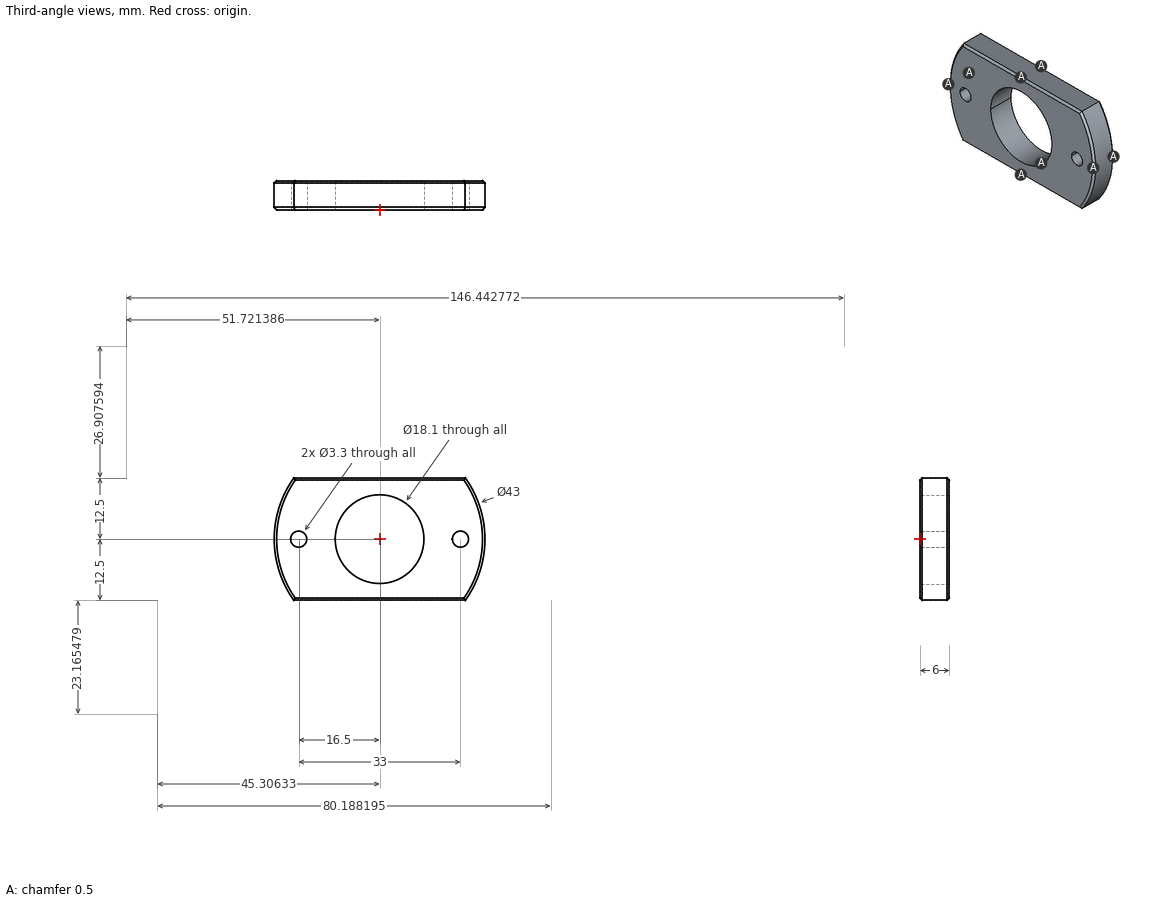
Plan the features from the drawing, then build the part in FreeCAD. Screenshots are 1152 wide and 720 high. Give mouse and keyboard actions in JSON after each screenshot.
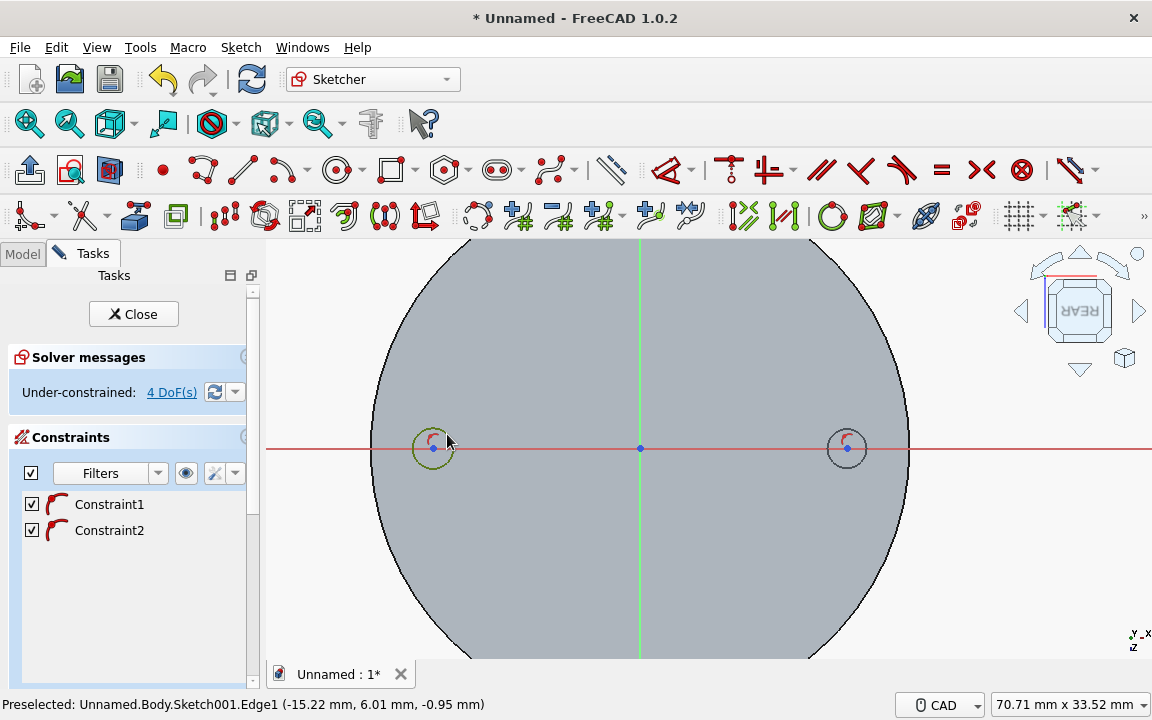
{"action": "left_click", "coordinate": [861, 435]}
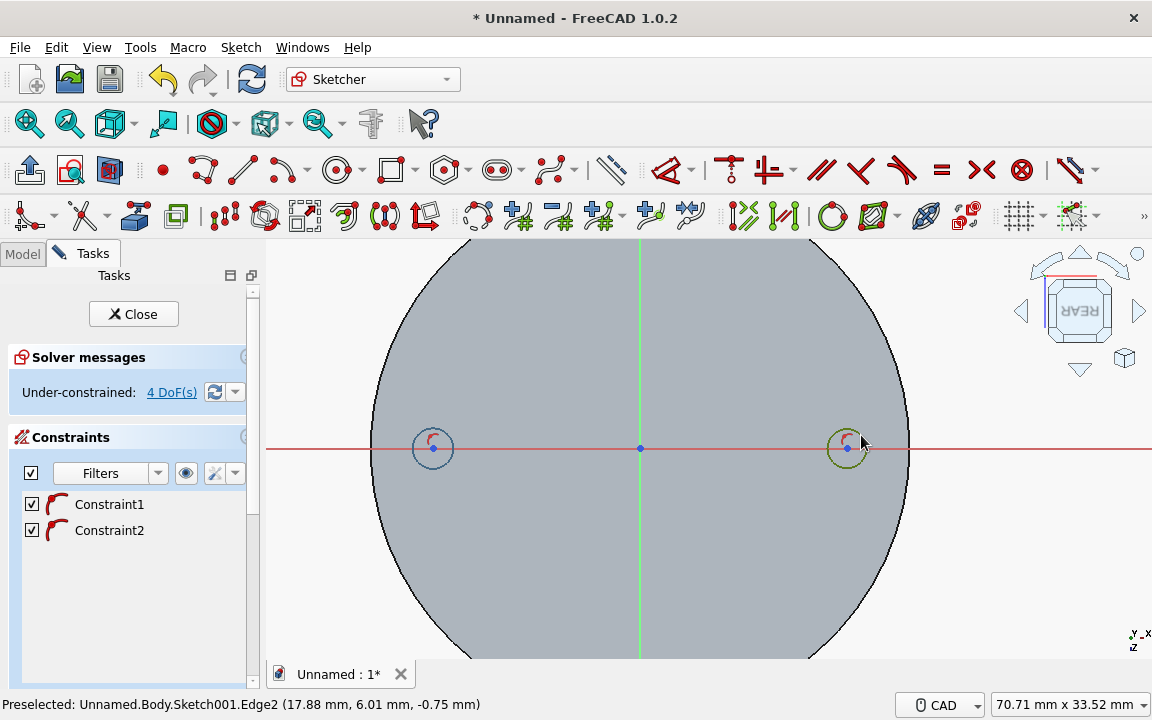
{"action": "left_click", "coordinate": [942, 170]}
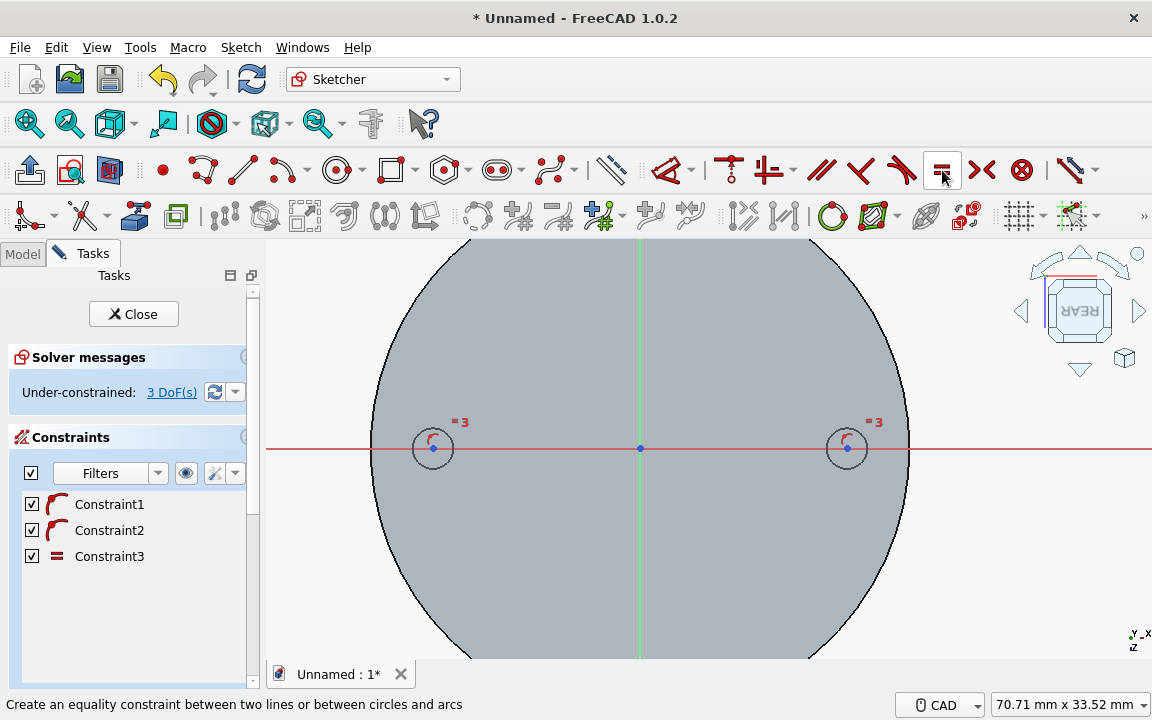
{"action": "left_click", "coordinate": [666, 170]}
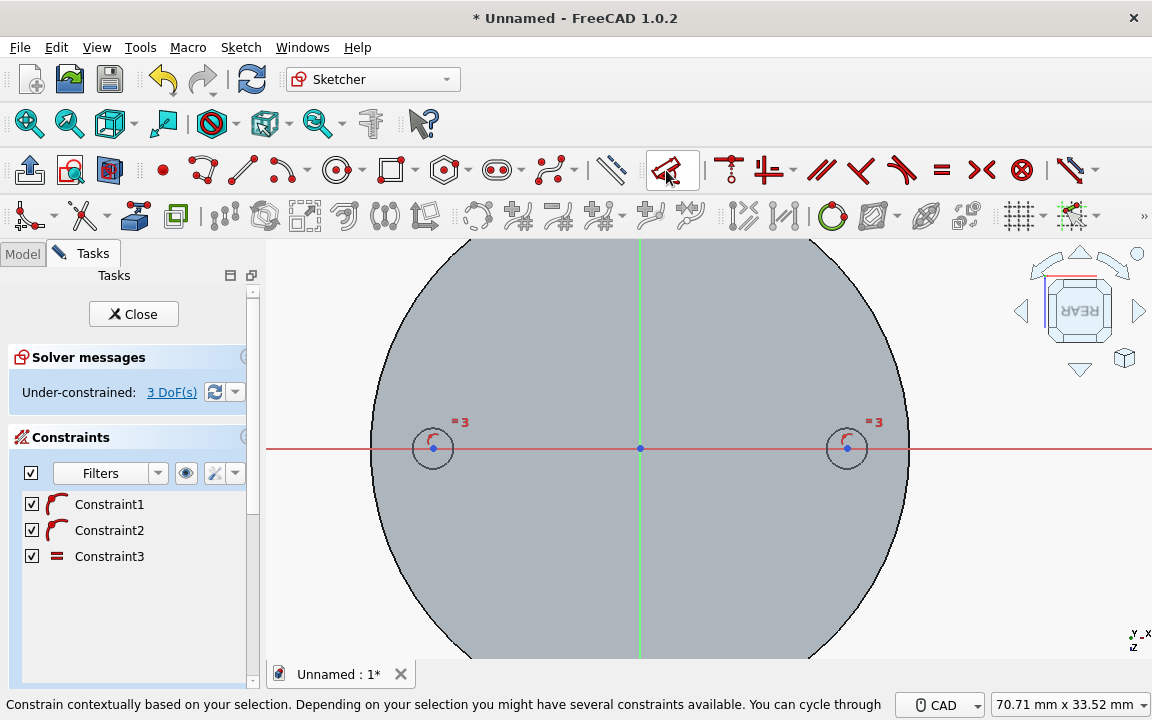
{"action": "left_click", "coordinate": [447, 434]}
{"action": "left_click", "coordinate": [469, 411]}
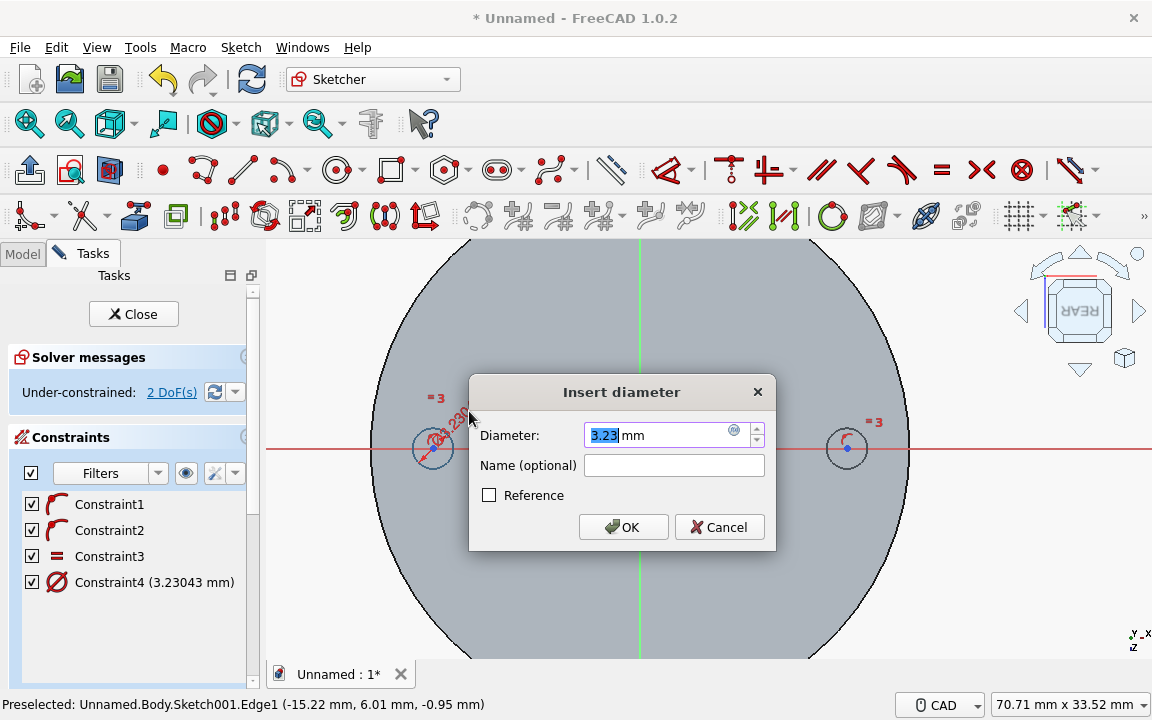
{"action": "type", "text": "3.3"}
{"action": "key", "text": "Return"}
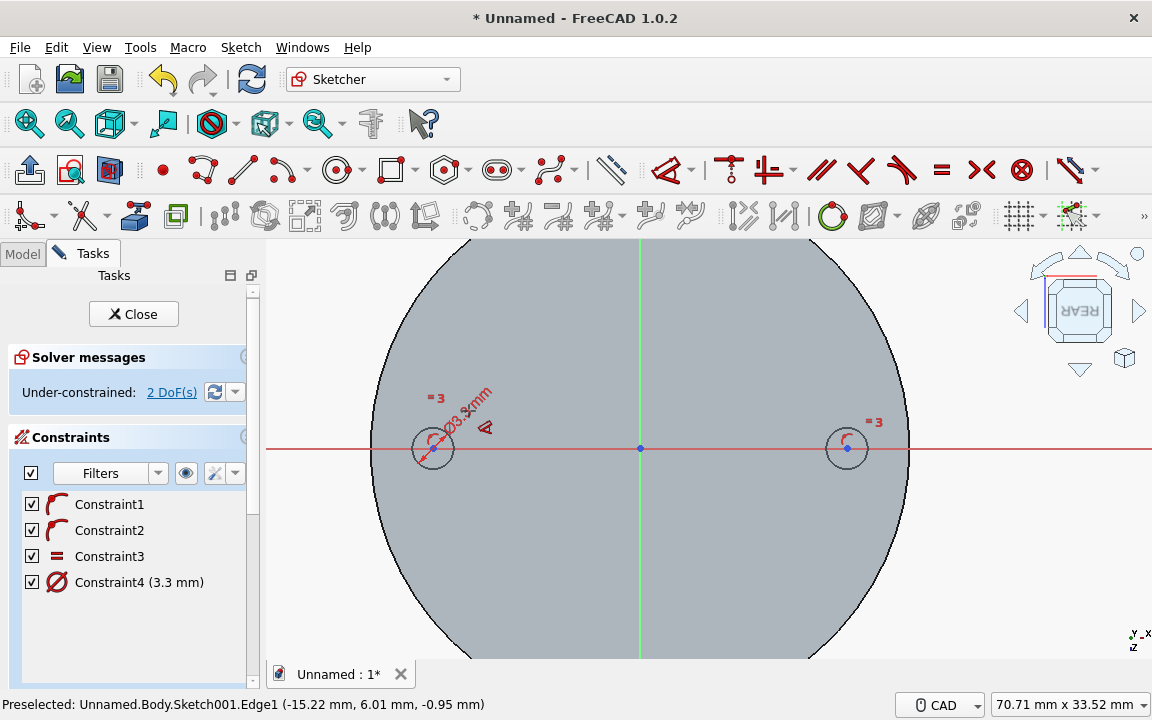
{"action": "left_click", "coordinate": [433, 449]}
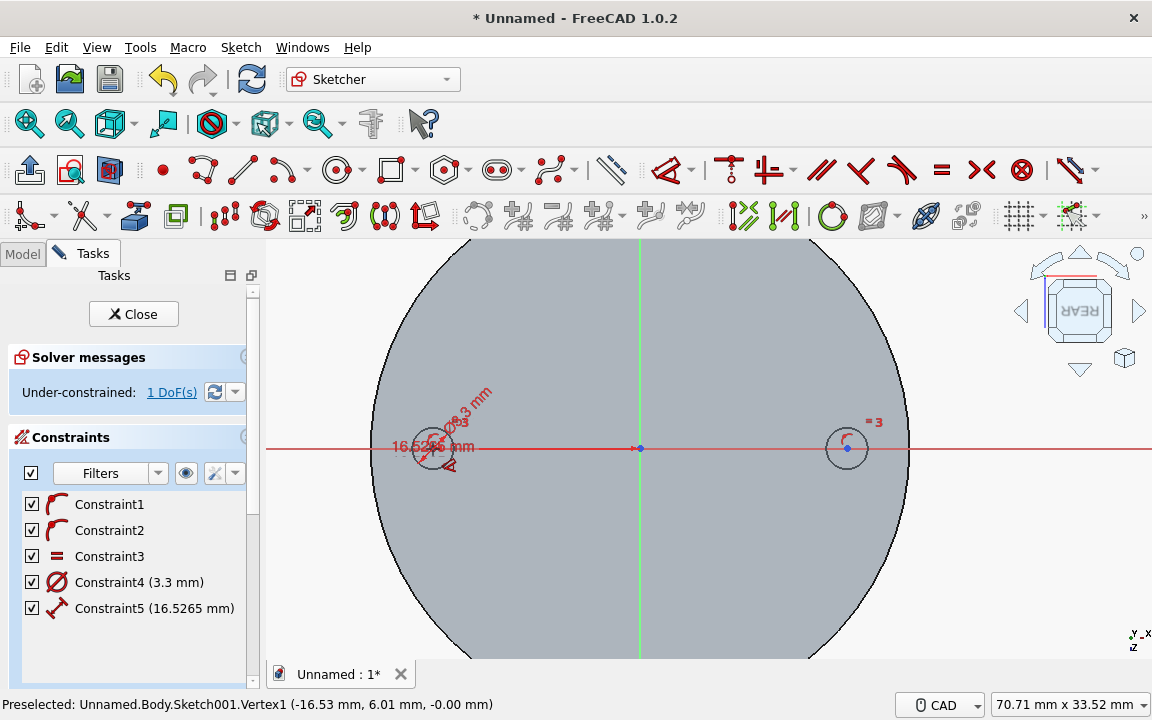
{"action": "left_click", "coordinate": [847, 449]}
{"action": "left_click", "coordinate": [545, 483]}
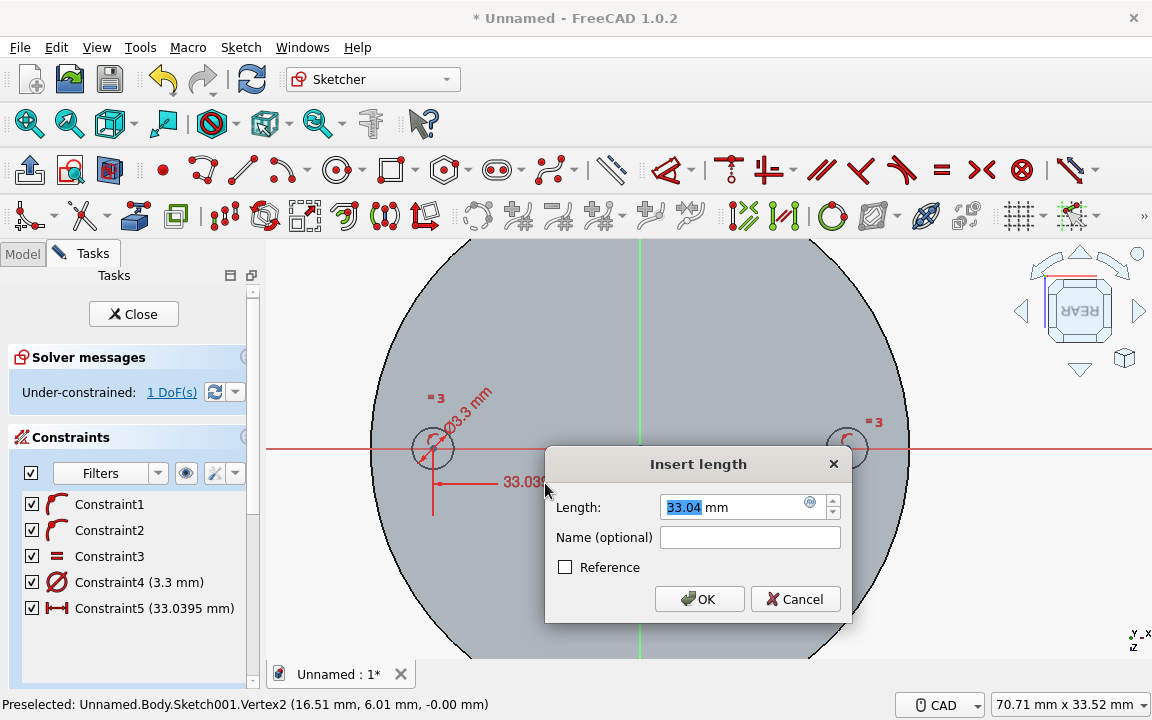
{"action": "type", "text": "33"}
{"action": "key", "text": "Return"}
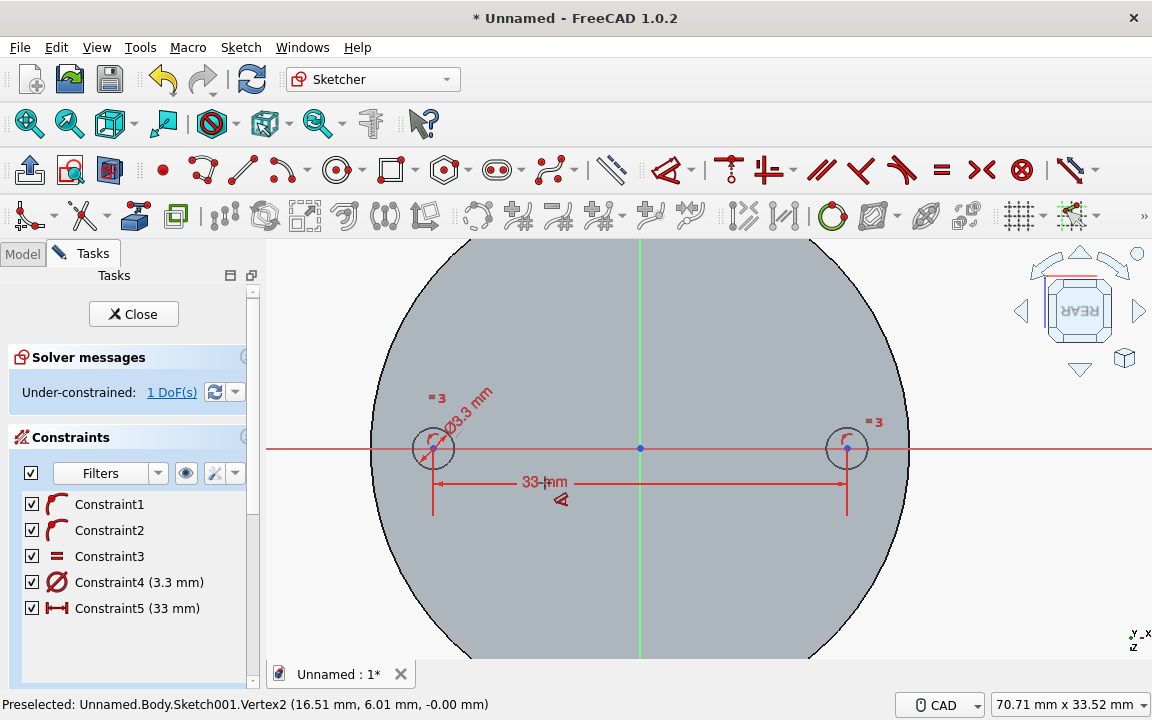
{"action": "left_click", "coordinate": [433, 449]}
{"action": "left_click", "coordinate": [464, 483]}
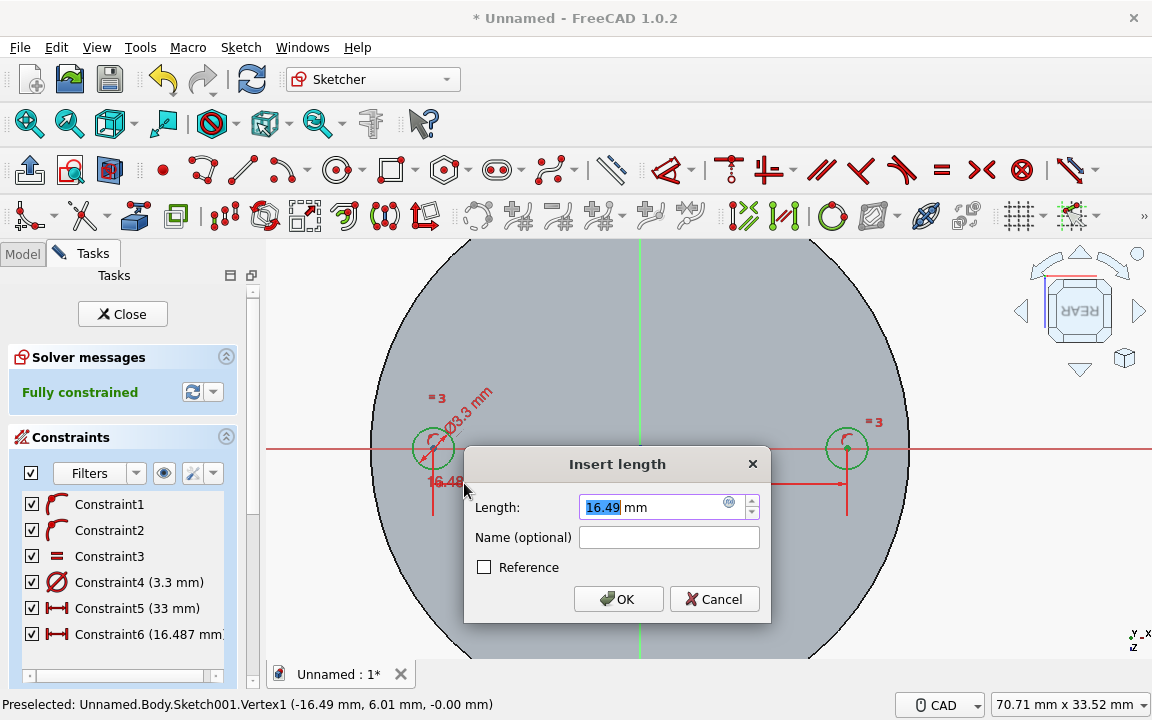
{"action": "type", "text": "16.5"}
{"action": "key", "text": "Return"}
{"action": "key", "text": "Escape"}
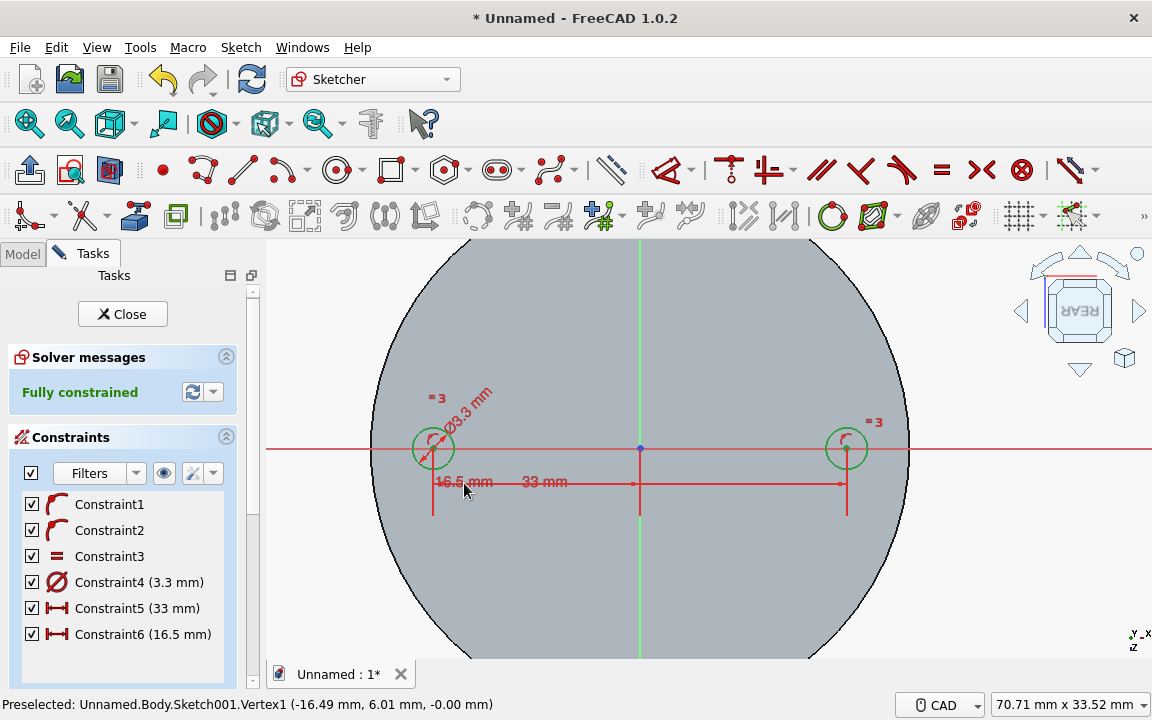
{"action": "left_click", "coordinate": [123, 314]}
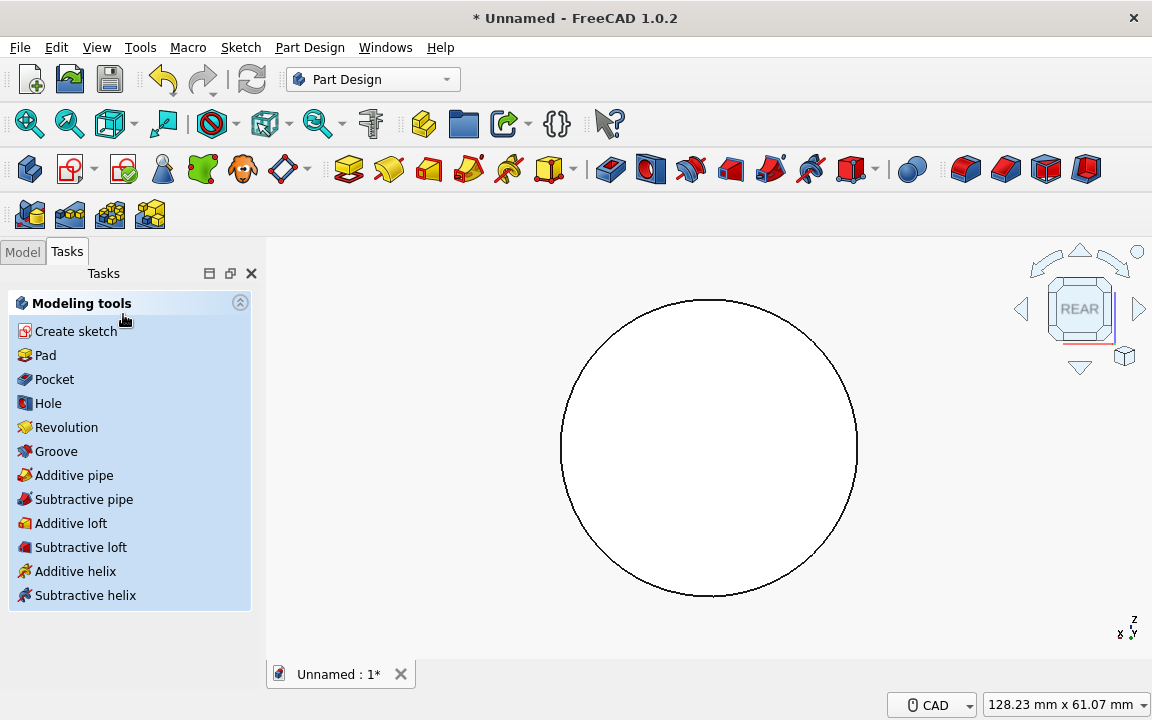
{"action": "left_click", "coordinate": [652, 170]}